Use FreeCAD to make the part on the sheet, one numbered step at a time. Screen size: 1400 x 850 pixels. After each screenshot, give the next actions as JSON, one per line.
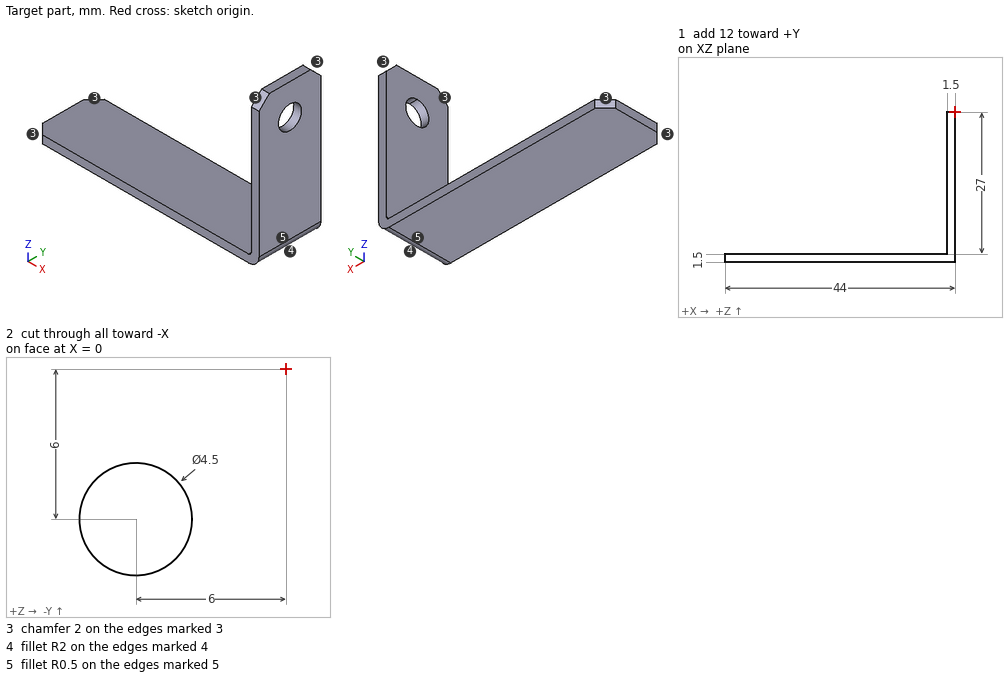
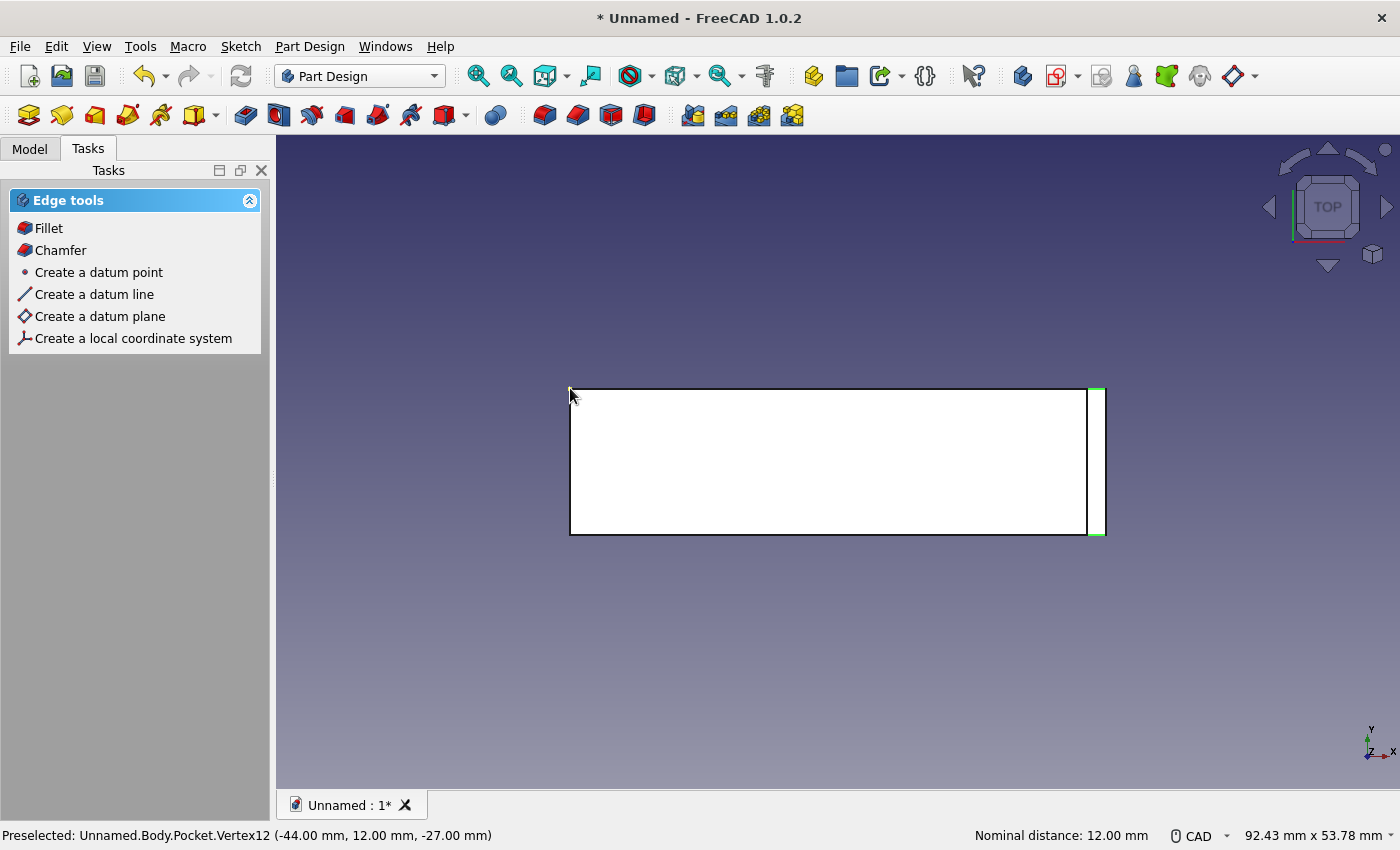
{"action": "key", "text": "1"}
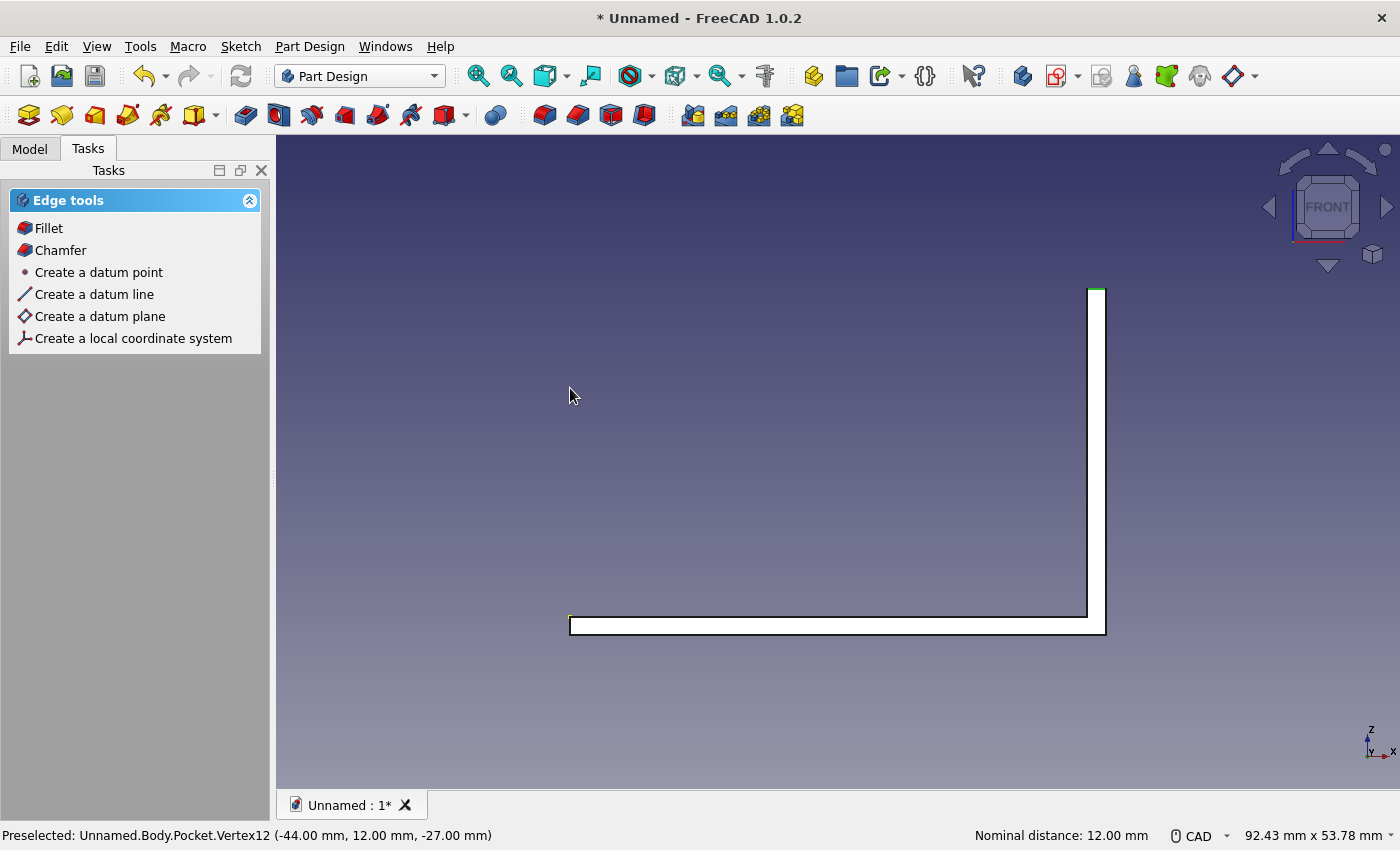
{"action": "left_click", "coordinate": [570, 625], "text": "ctrl"}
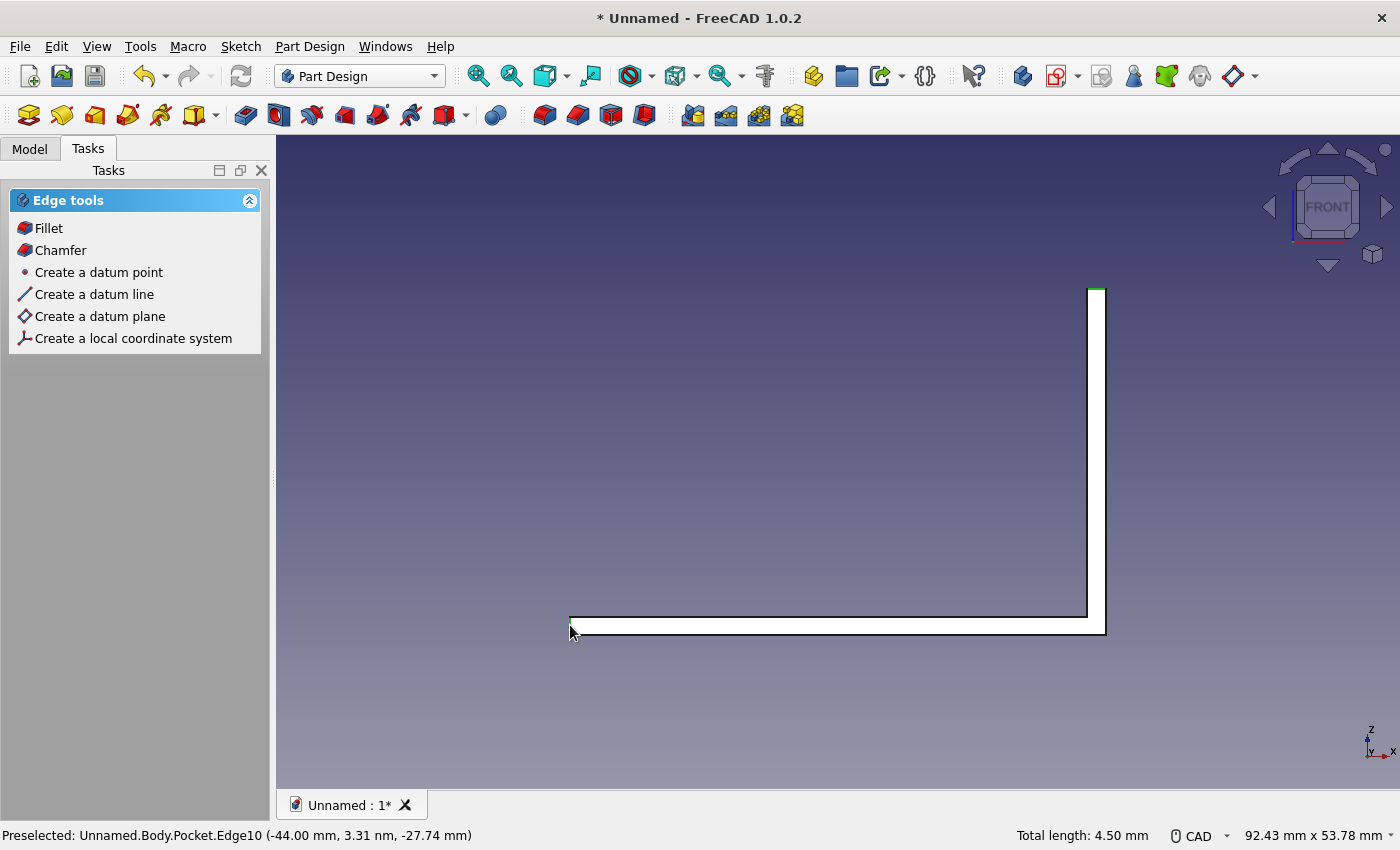
{"action": "scroll", "coordinate": [570, 625], "scroll_direction": "up", "scroll_amount": 4}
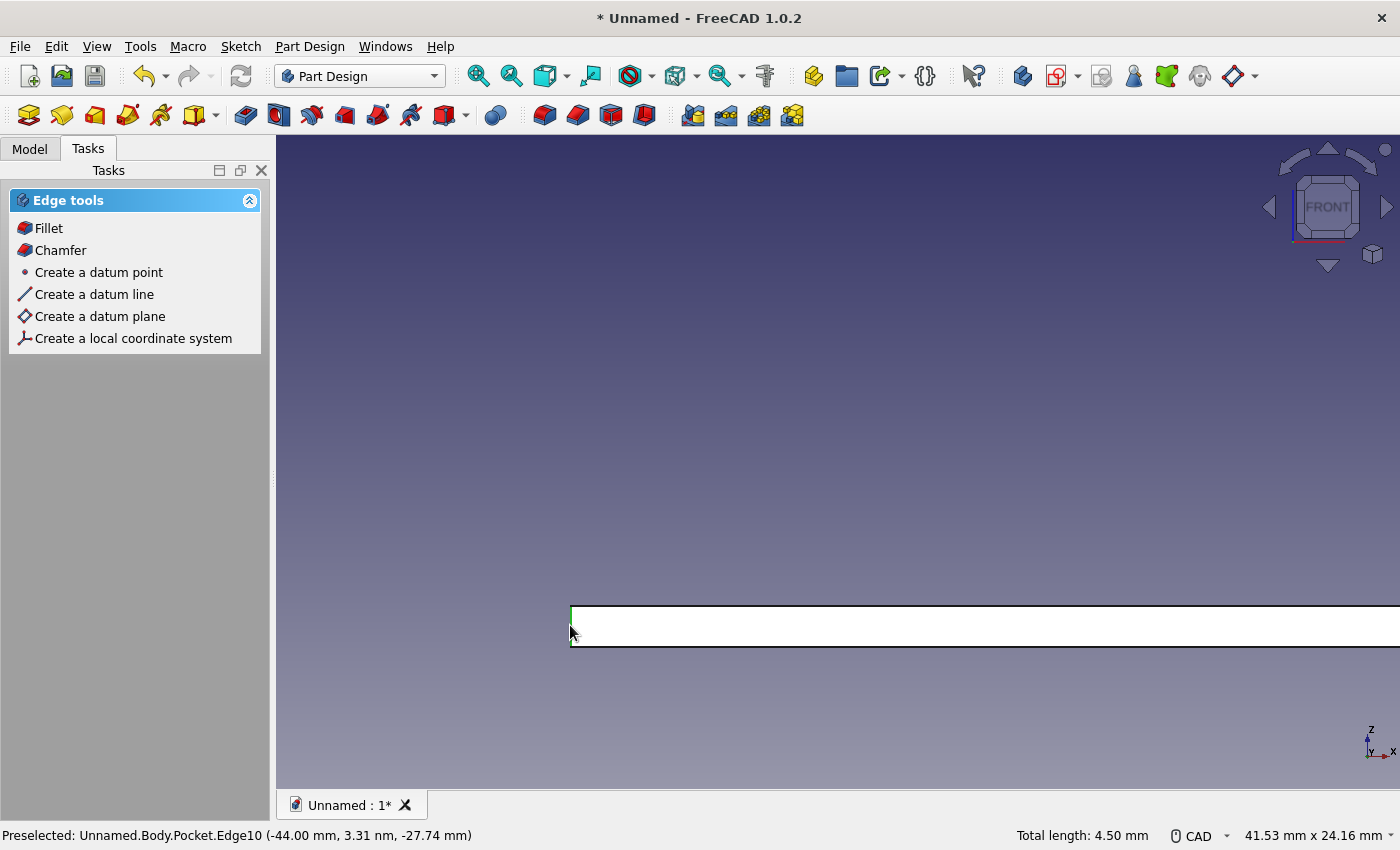
{"action": "key", "text": "v f"}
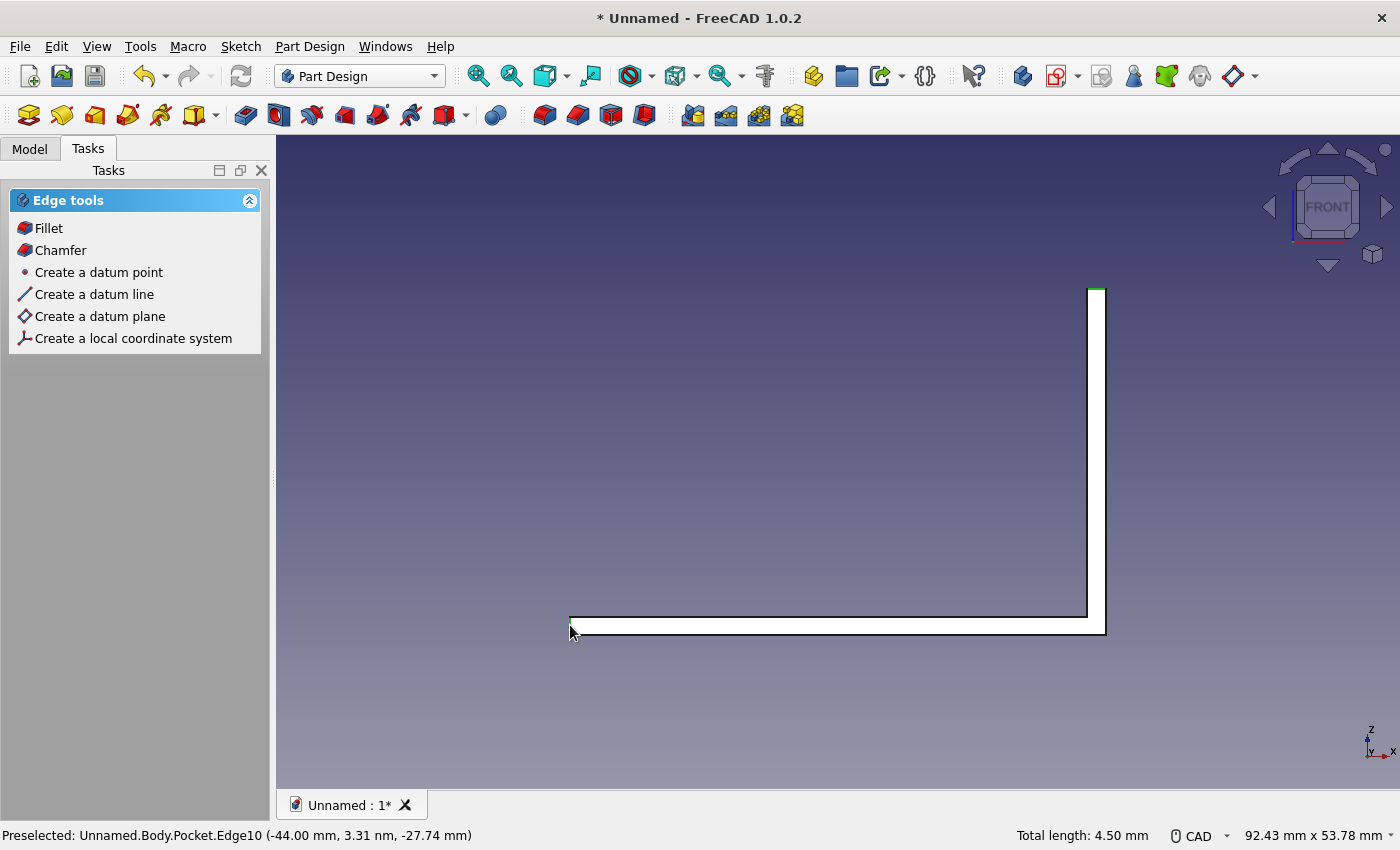
{"action": "key", "text": "3"}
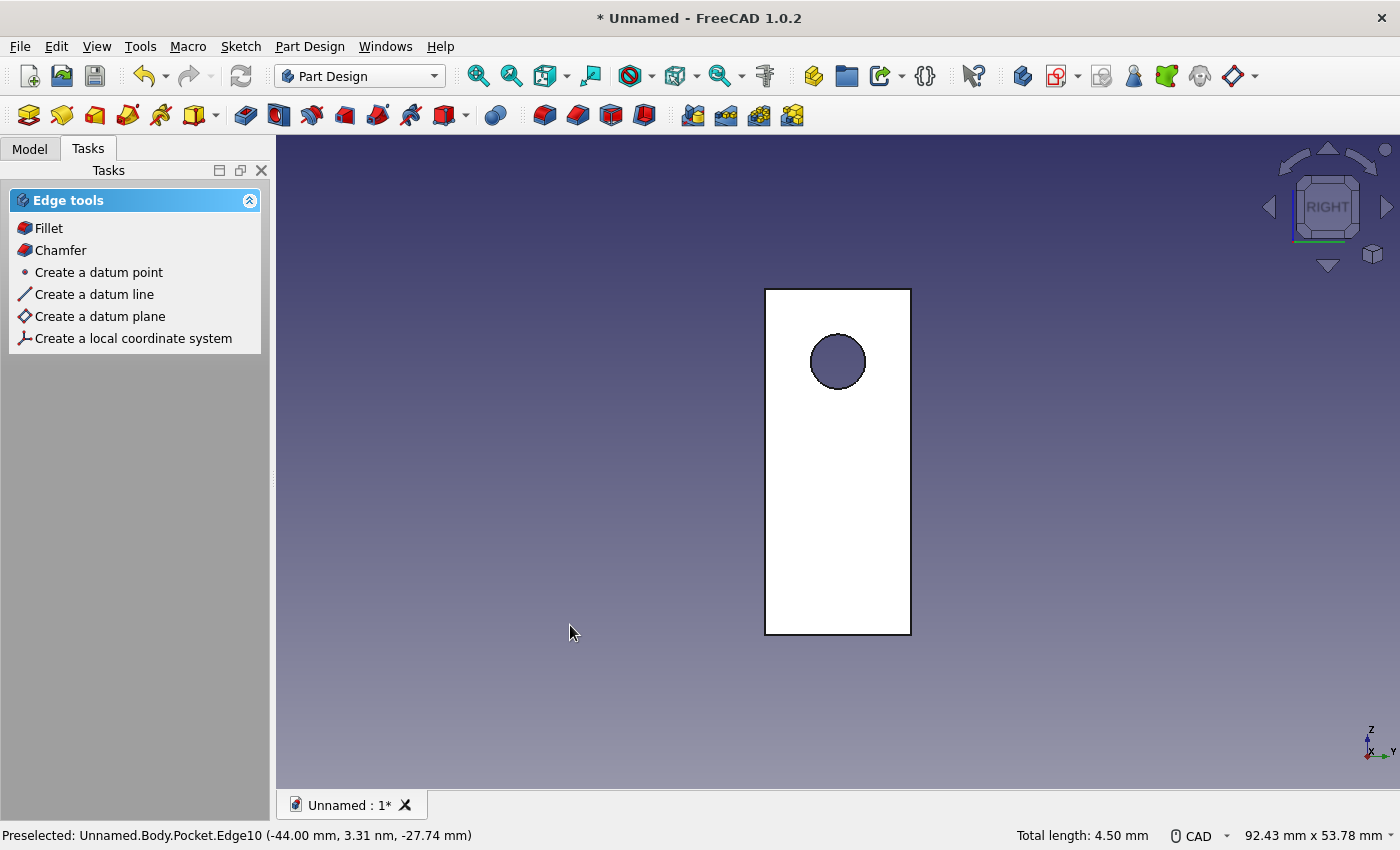
{"action": "scroll", "coordinate": [911, 625], "scroll_direction": "up", "scroll_amount": 4}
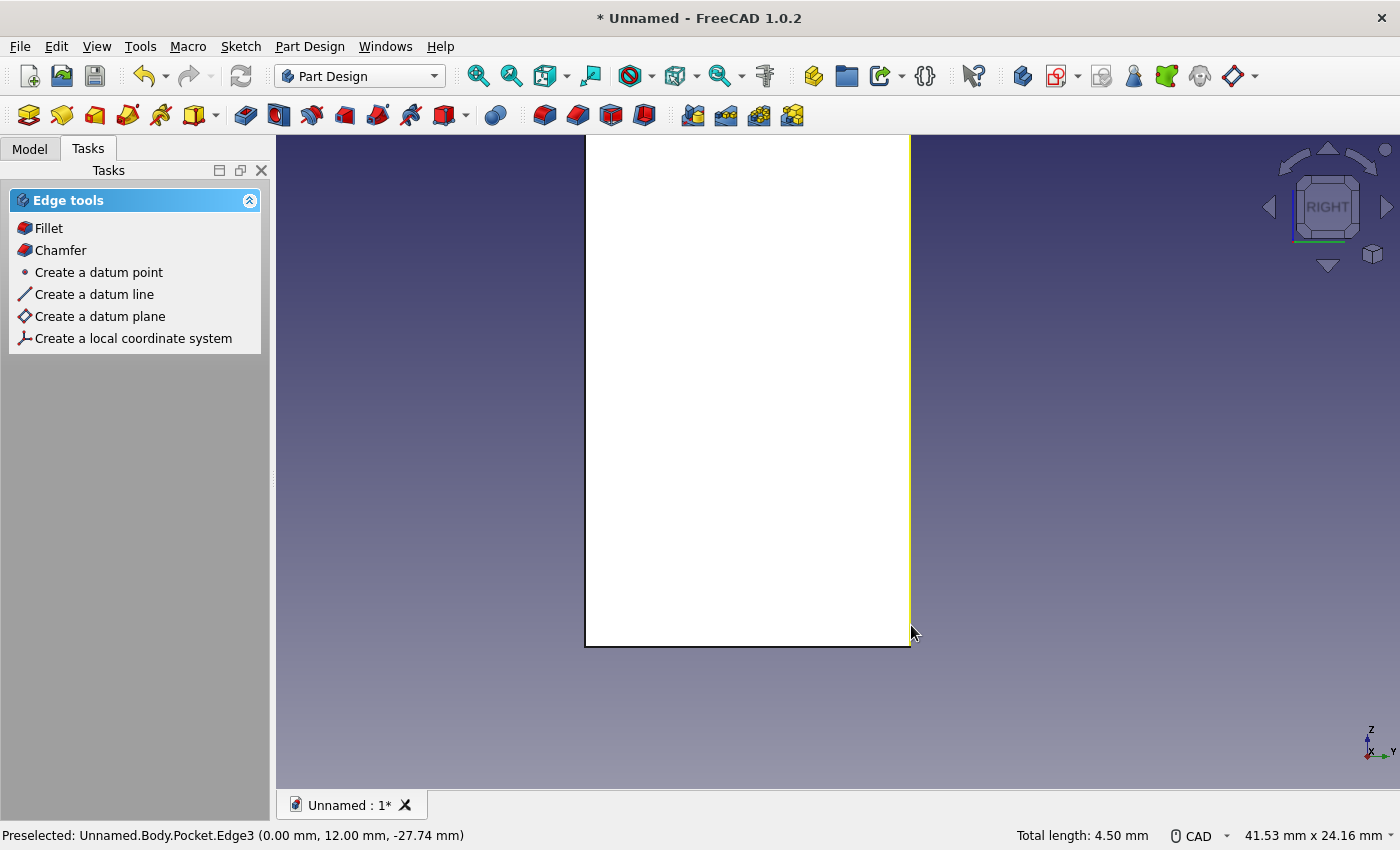
{"action": "left_click", "coordinate": [479, 76]}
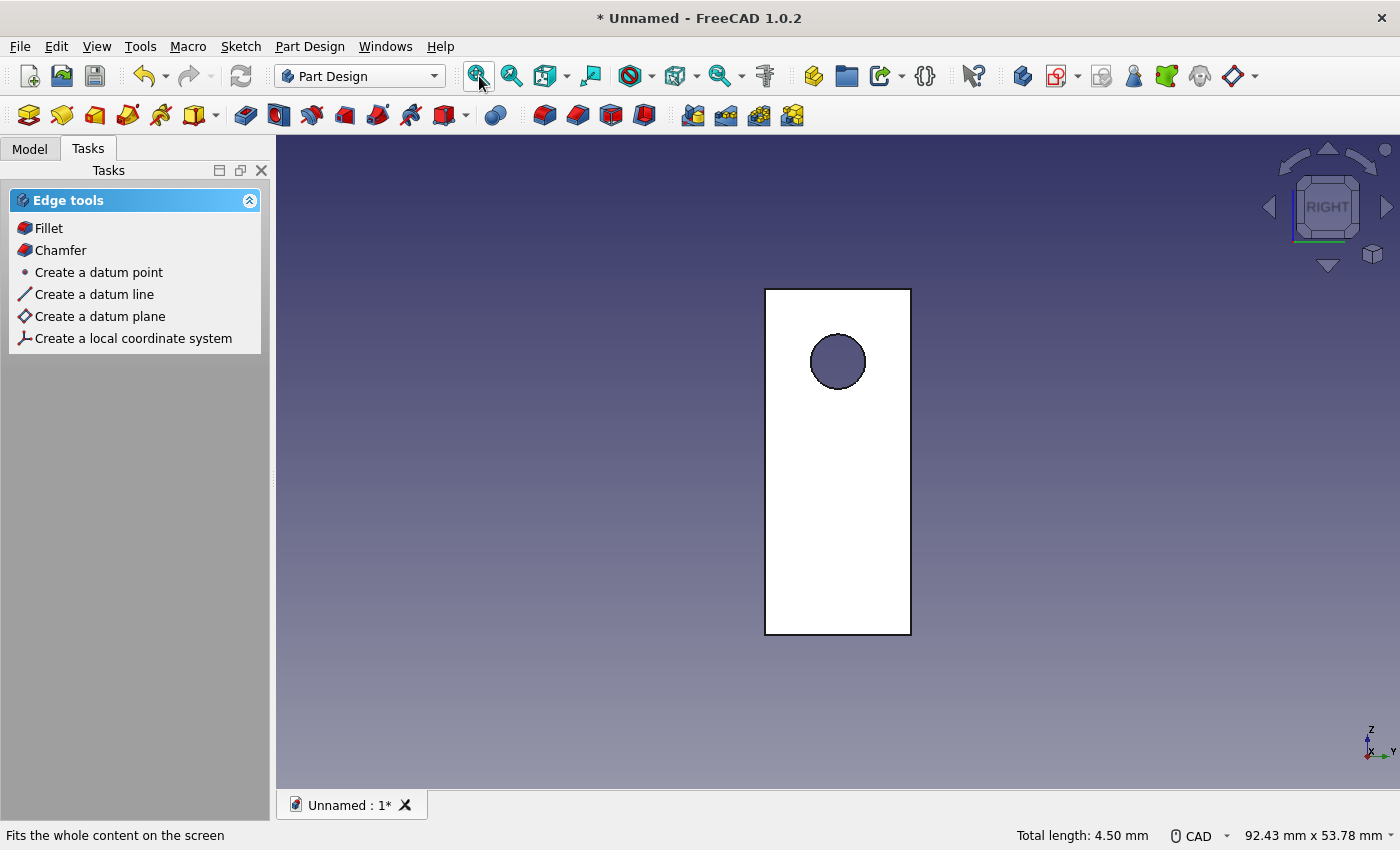
{"action": "key", "text": "5"}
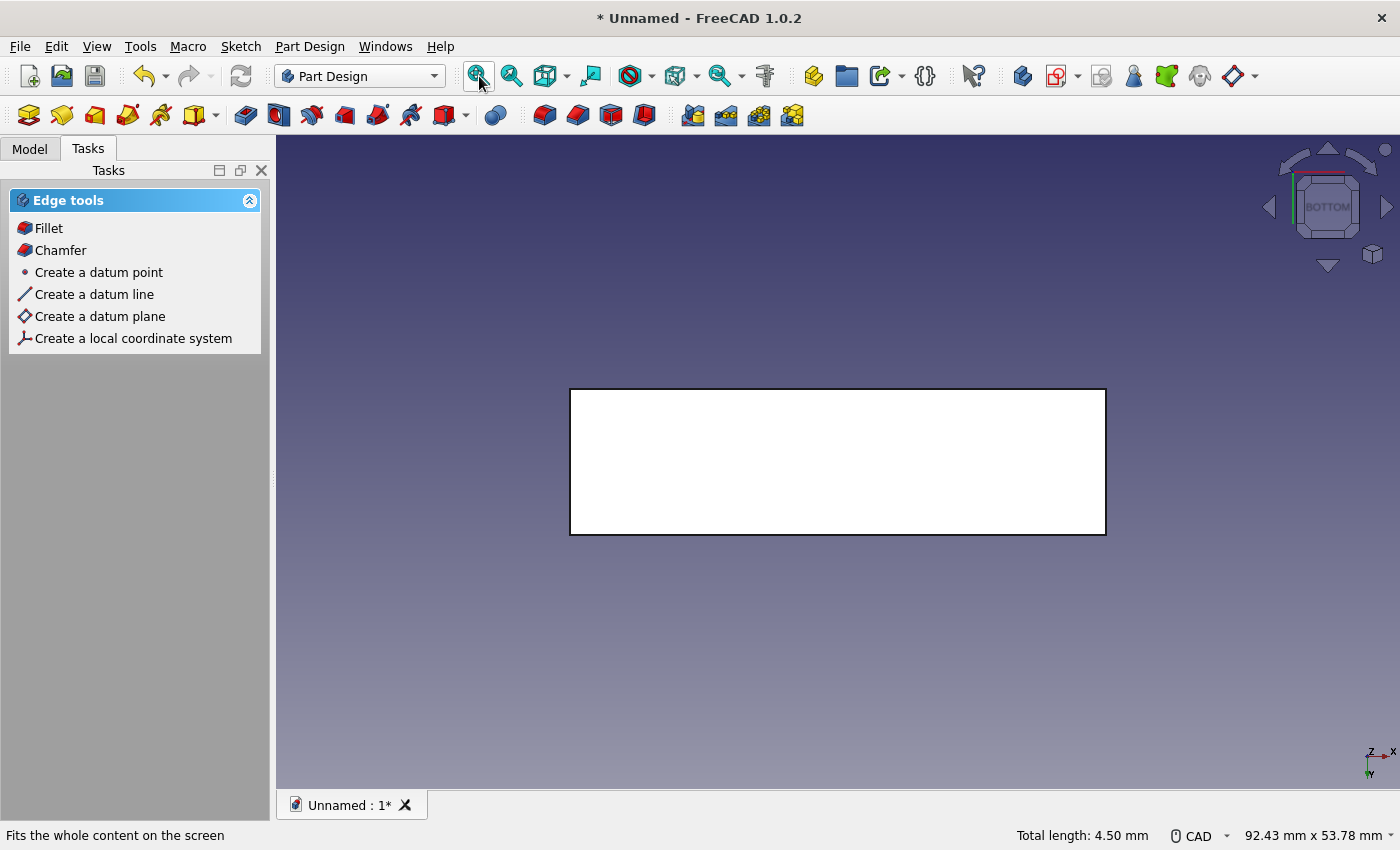
{"action": "scroll", "coordinate": [570, 534], "scroll_direction": "up", "scroll_amount": 4}